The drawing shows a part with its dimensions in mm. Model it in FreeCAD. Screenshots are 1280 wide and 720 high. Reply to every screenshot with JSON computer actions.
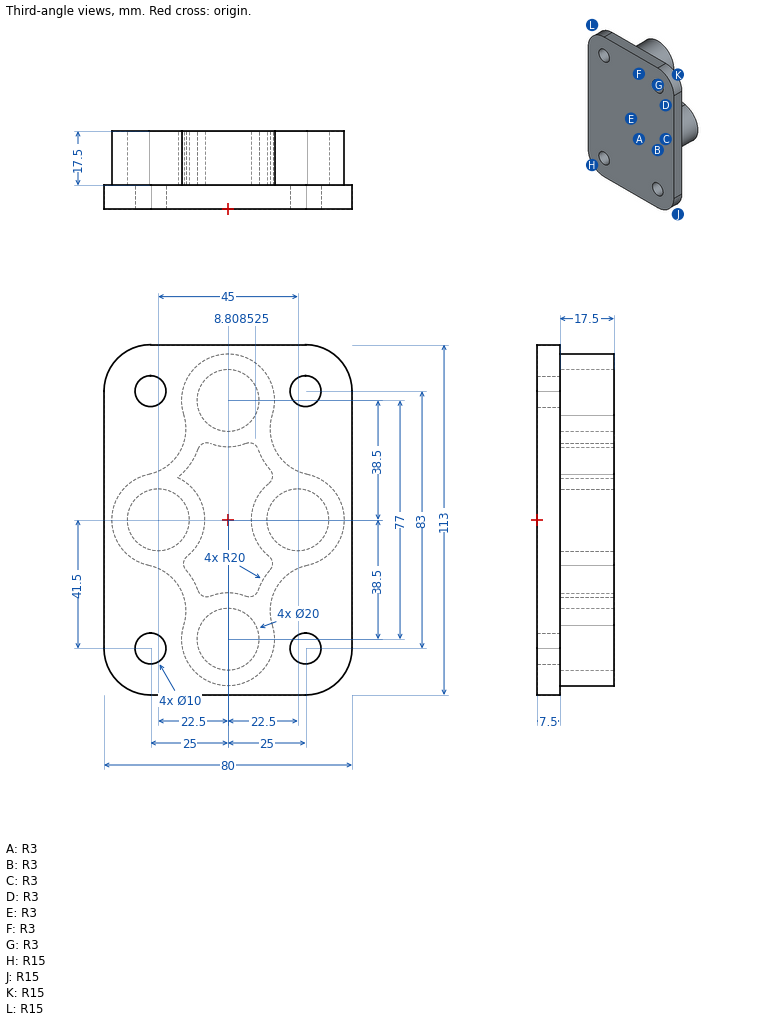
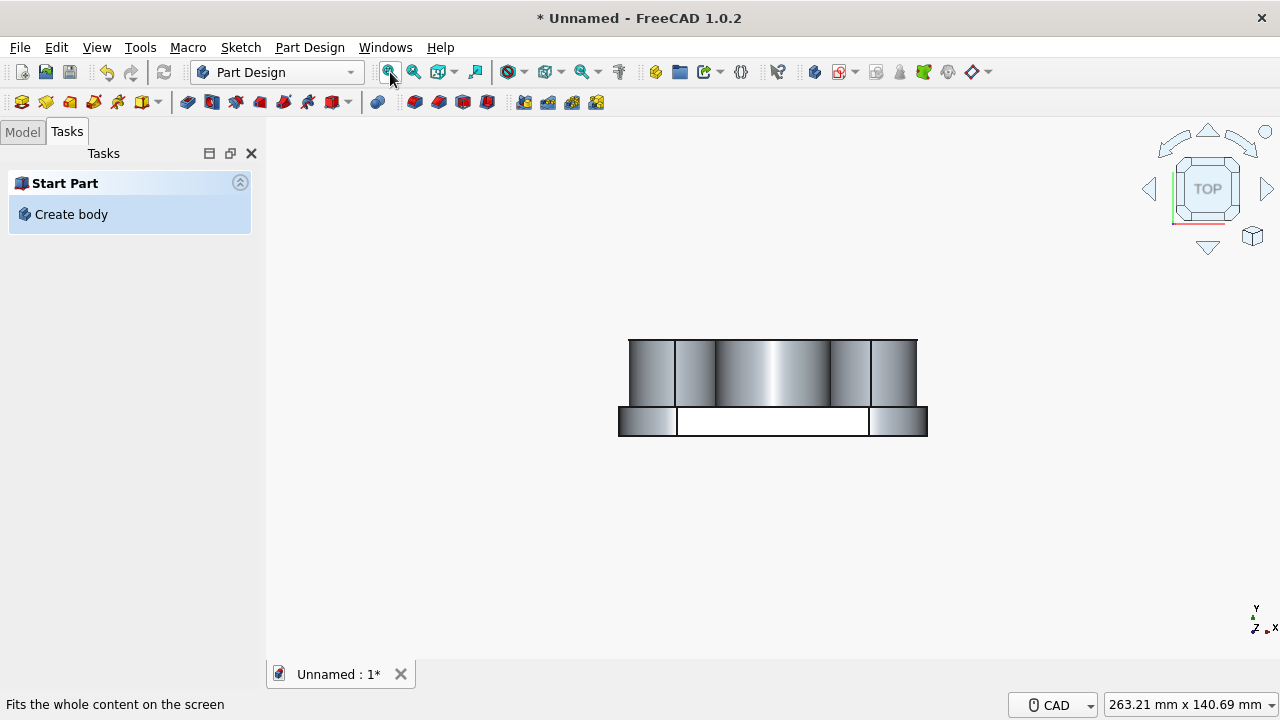
{"action": "key", "text": "4"}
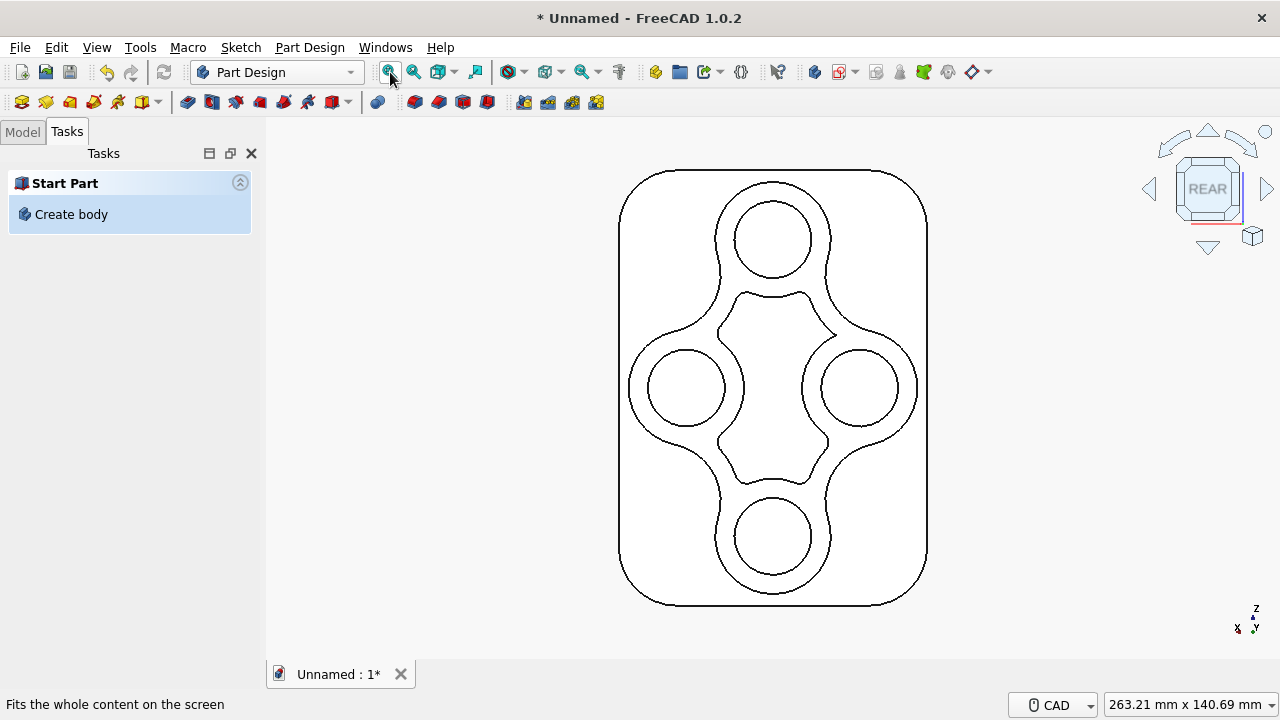
{"action": "left_click", "coordinate": [685, 511]}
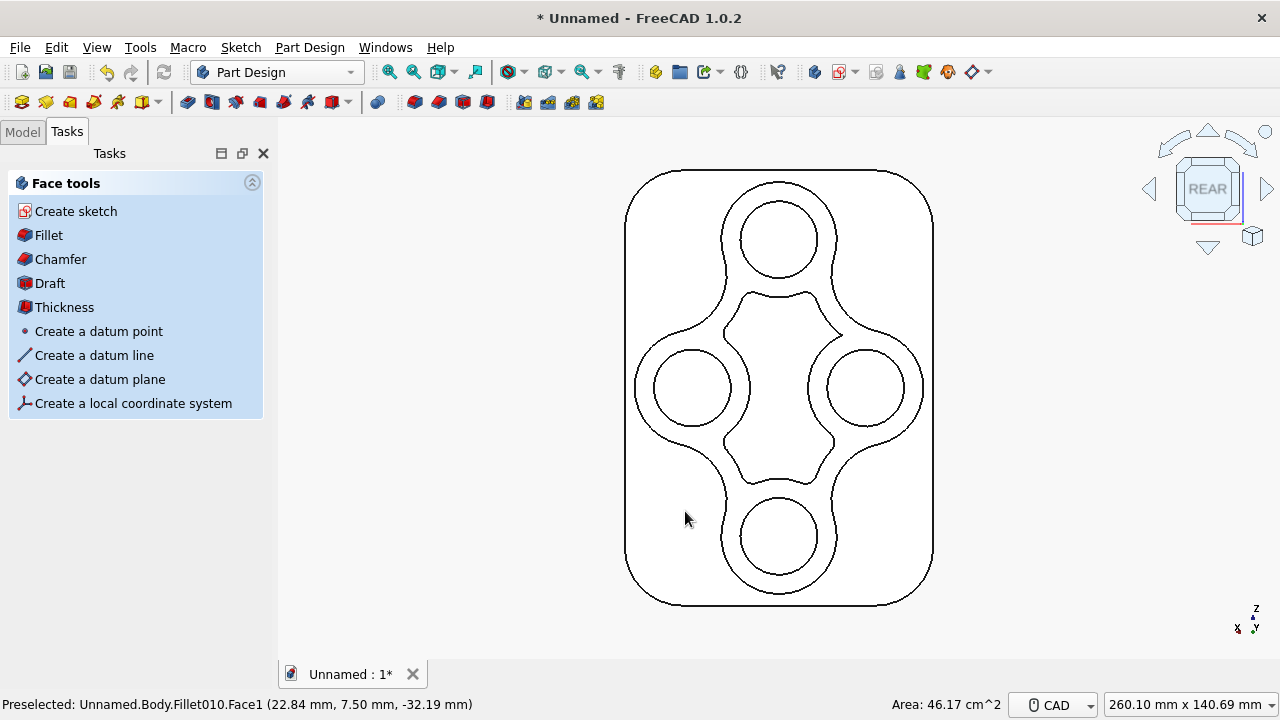
{"action": "left_click", "coordinate": [840, 72]}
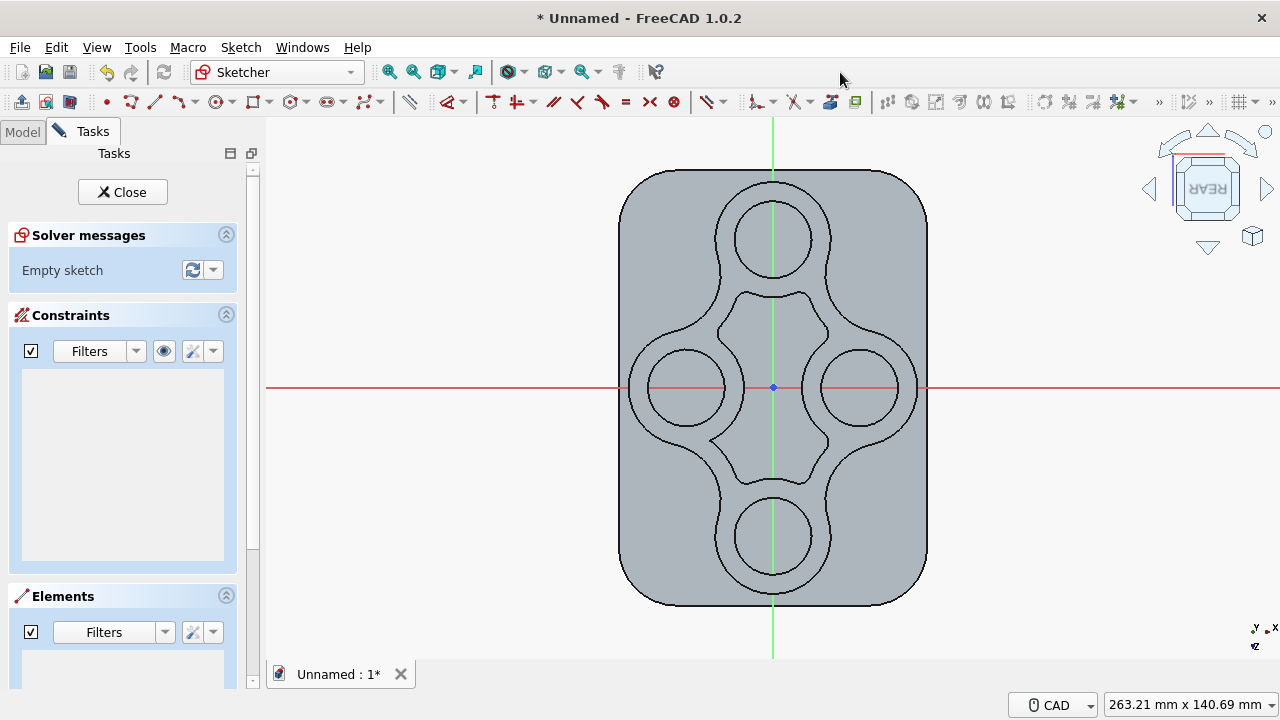
{"action": "key", "text": "g c"}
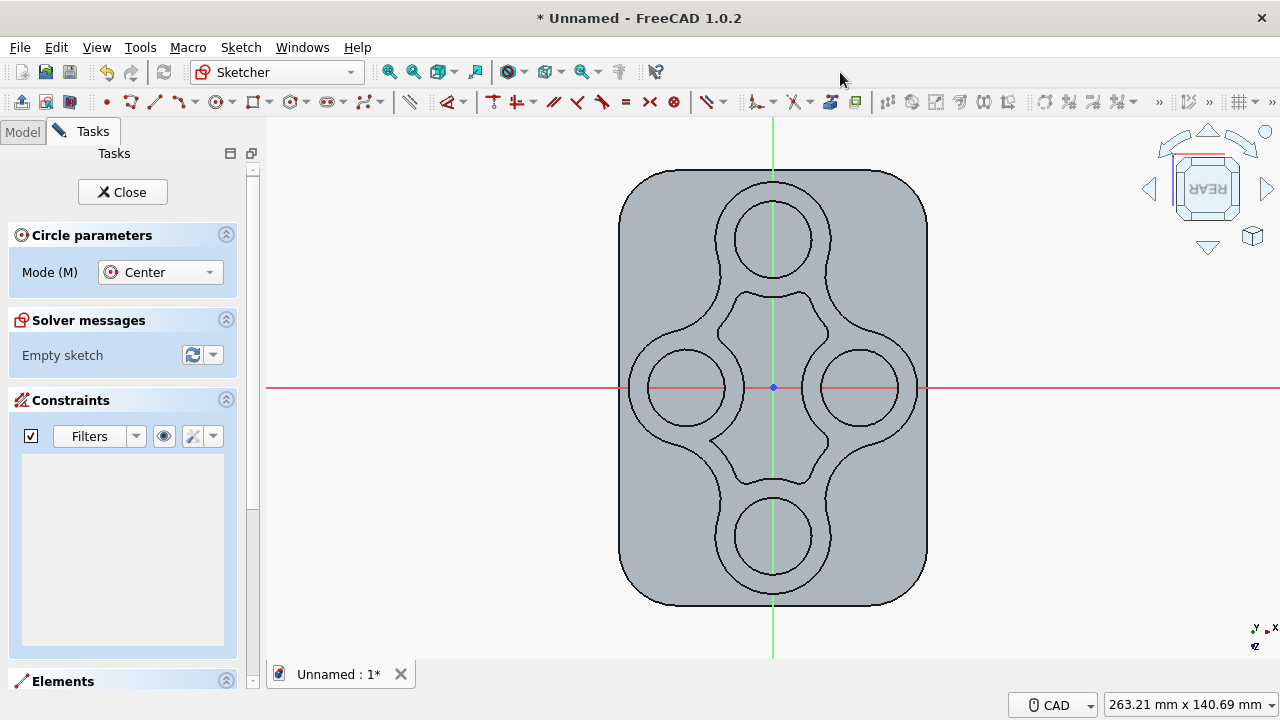
{"action": "left_click", "coordinate": [677, 228]}
{"action": "mouse_move", "coordinate": [690, 215]}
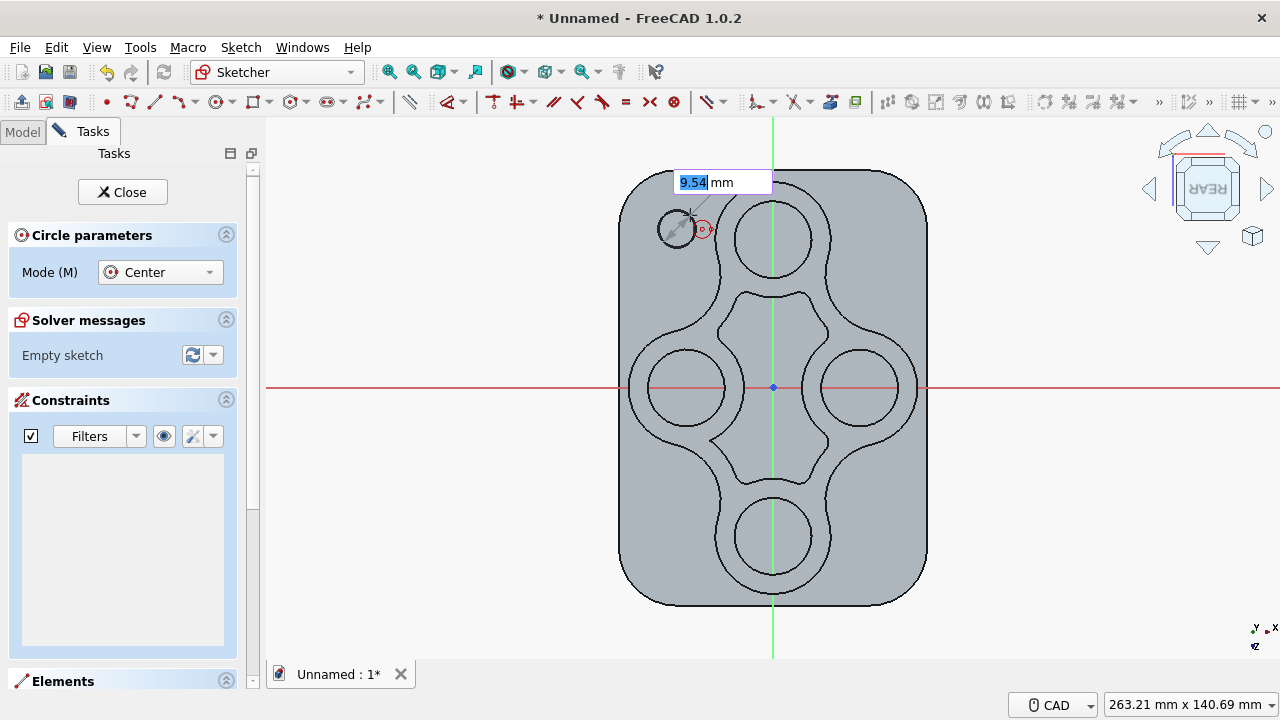
{"action": "type", "text": "10"}
{"action": "key", "text": "Return"}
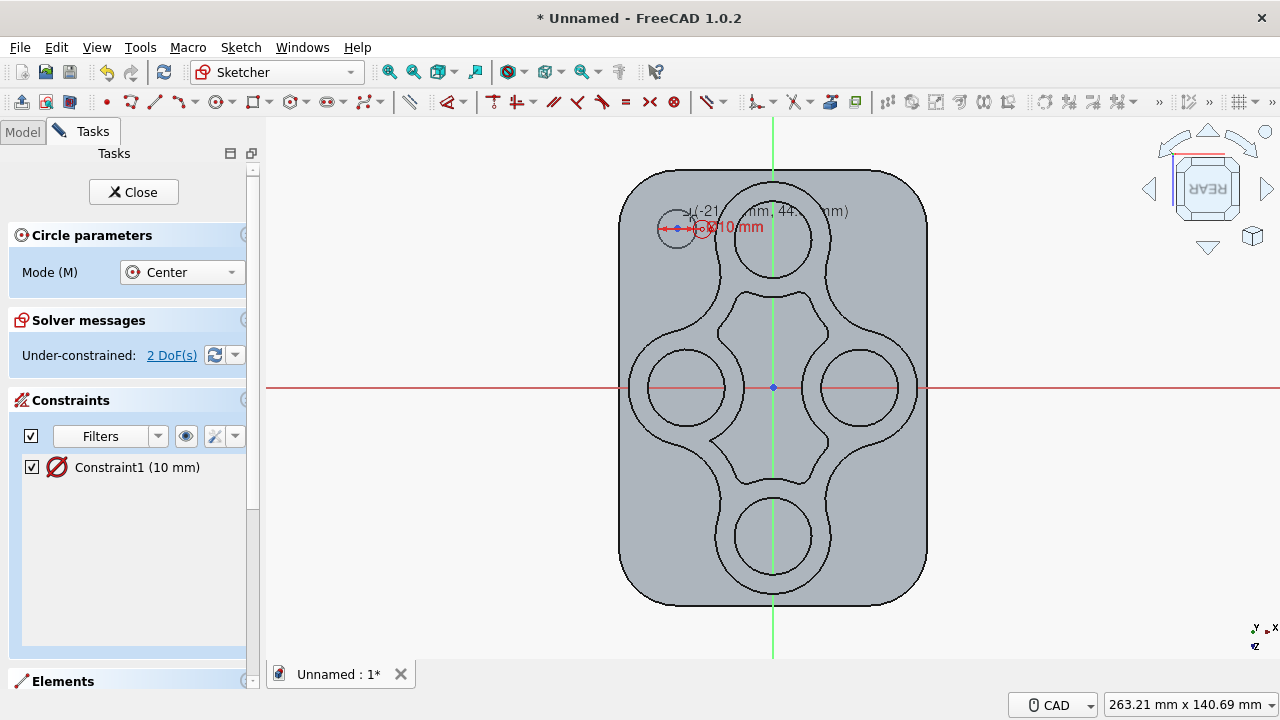
{"action": "left_click", "coordinate": [869, 228]}
{"action": "mouse_move", "coordinate": [883, 215]}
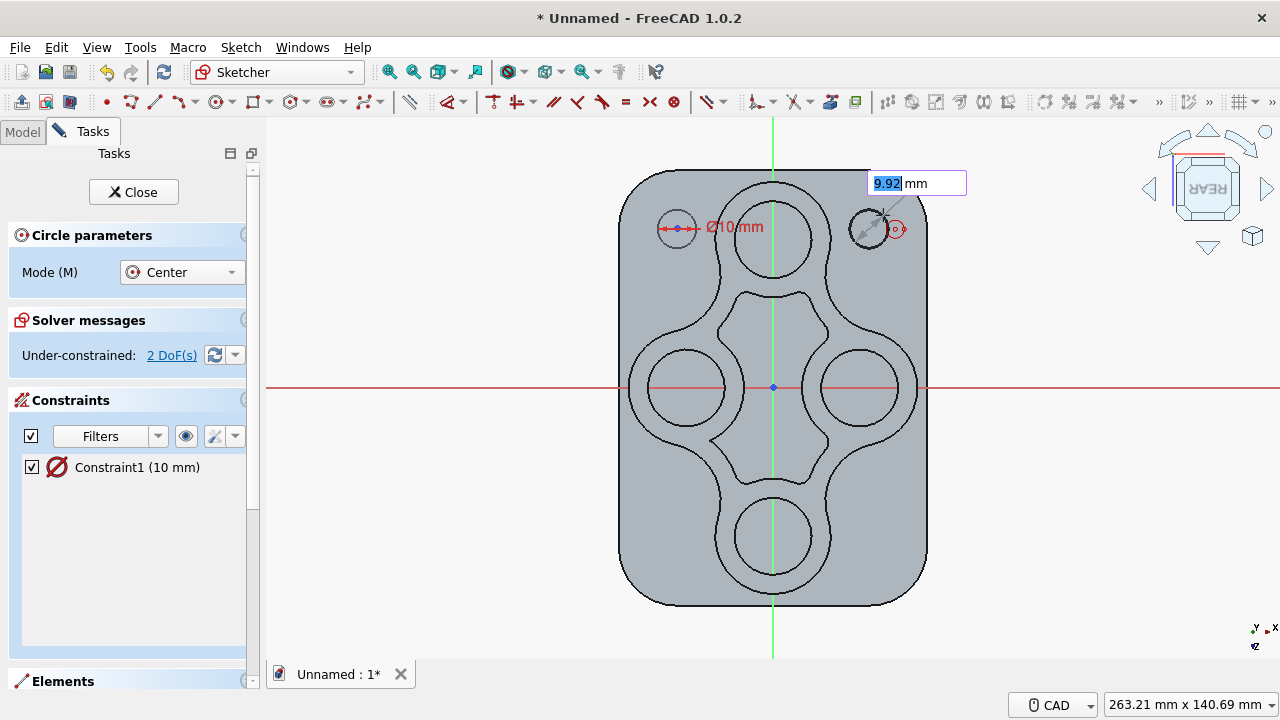
{"action": "type", "text": "10"}
{"action": "key", "text": "Return"}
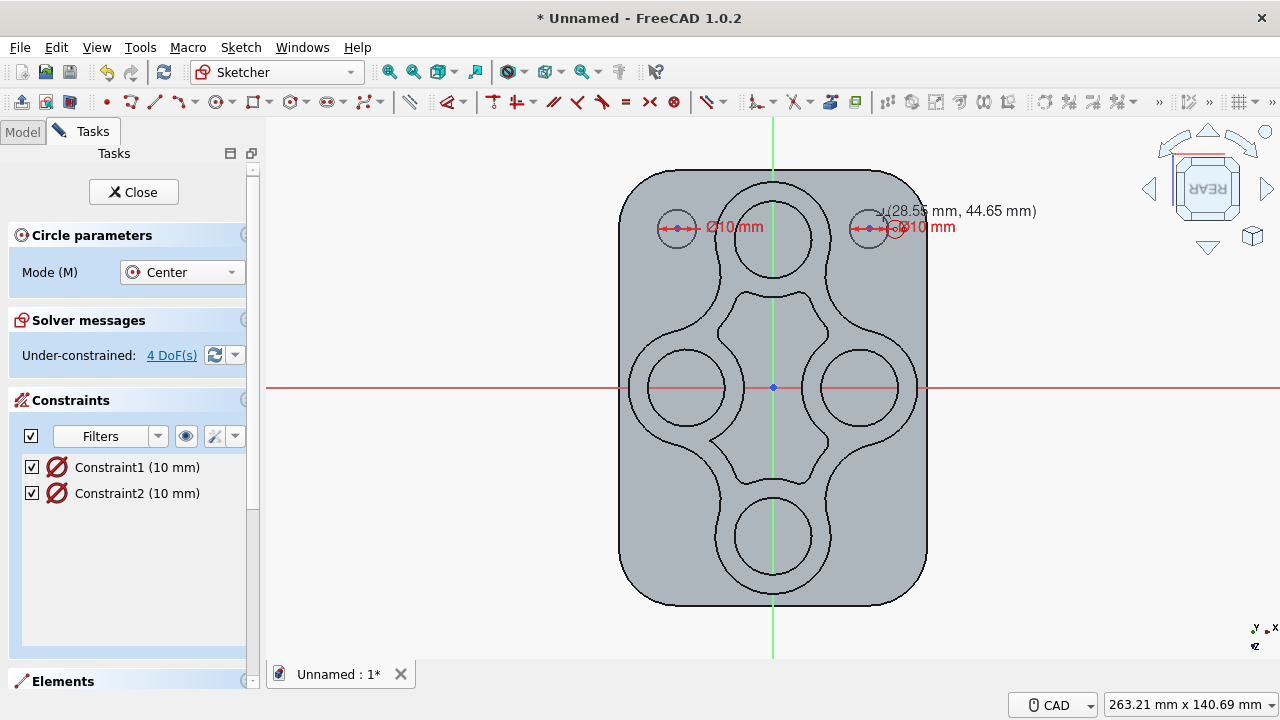
{"action": "left_click", "coordinate": [869, 548]}
{"action": "mouse_move", "coordinate": [883, 534]}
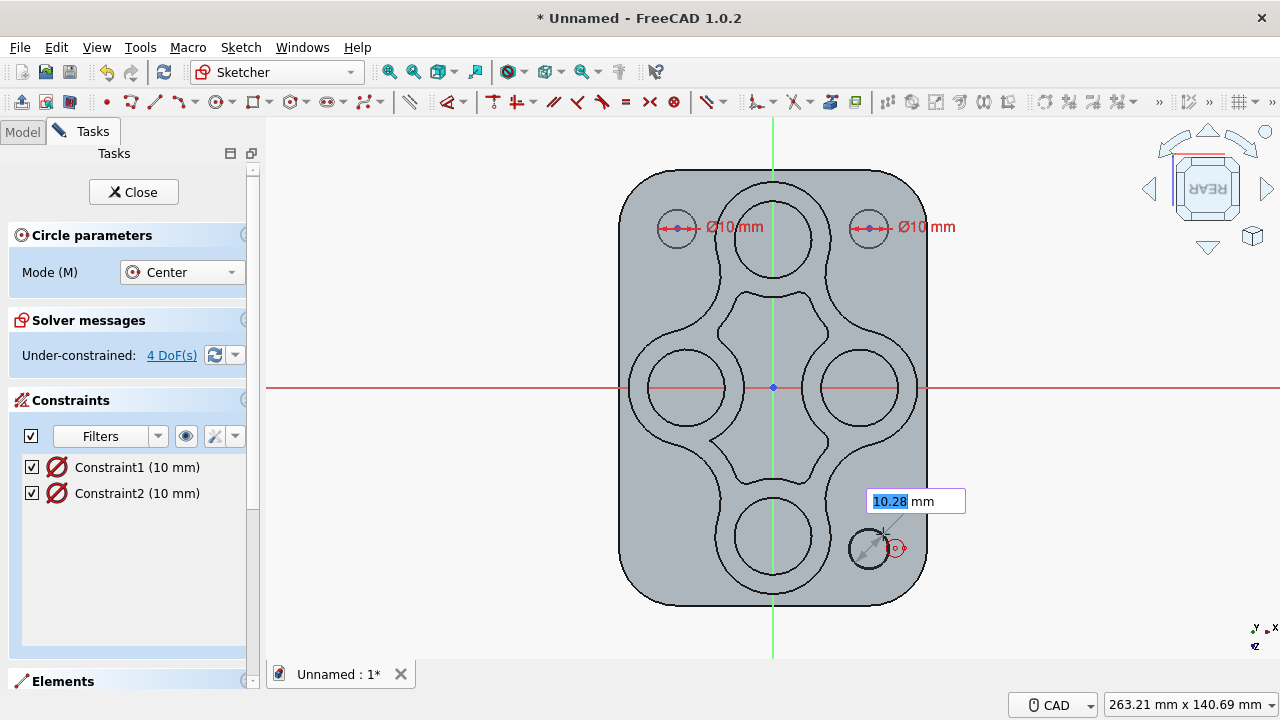
{"action": "type", "text": "10"}
{"action": "key", "text": "Return"}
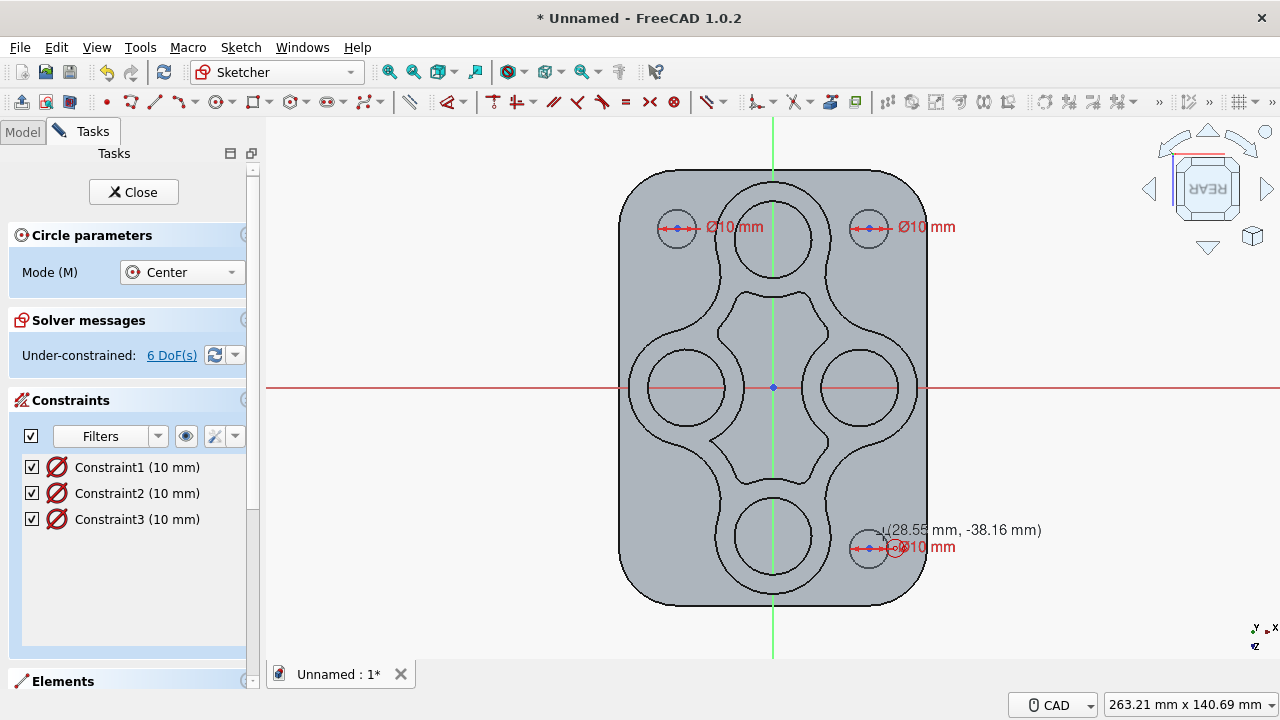
{"action": "left_click", "coordinate": [677, 548]}
{"action": "mouse_move", "coordinate": [690, 534]}